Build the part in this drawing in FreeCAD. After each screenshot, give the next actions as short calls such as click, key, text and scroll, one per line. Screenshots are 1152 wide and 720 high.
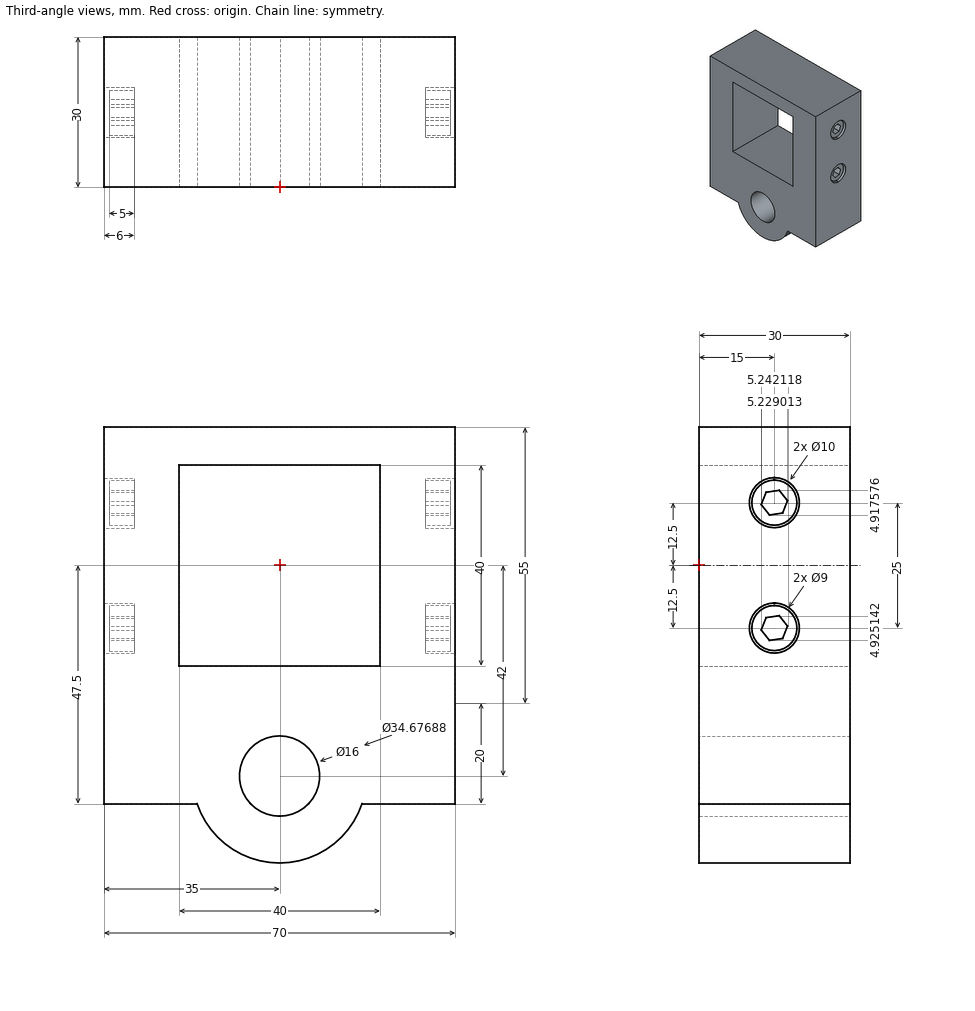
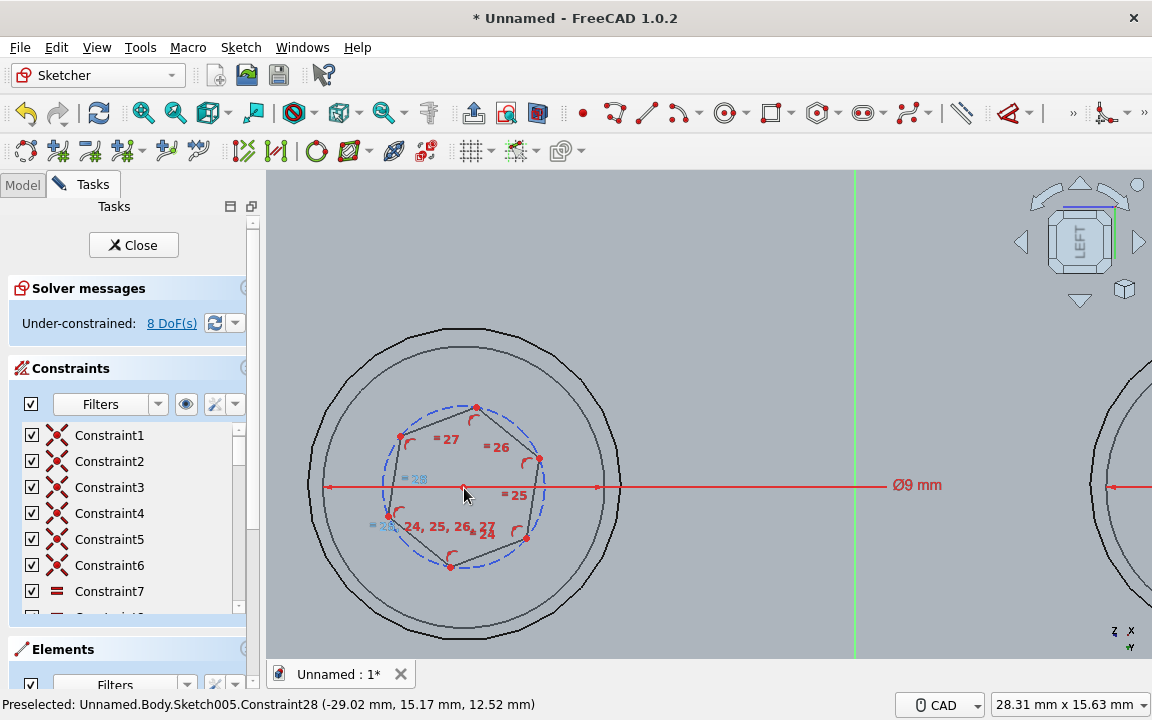
click(464, 487)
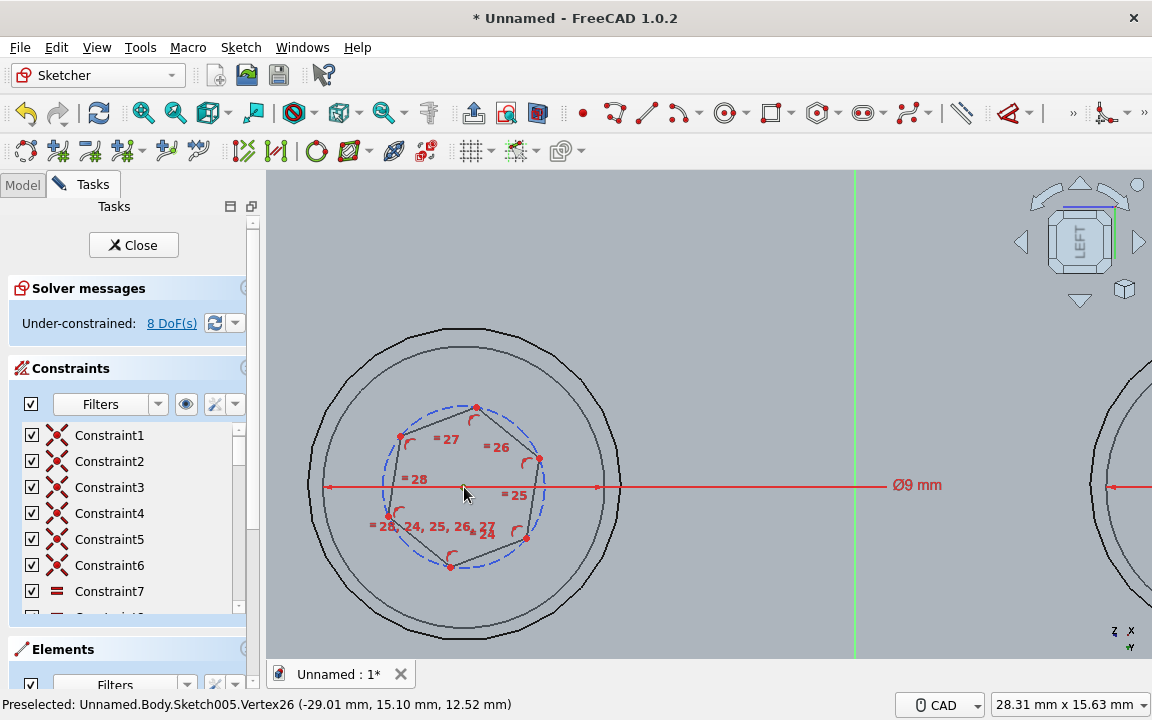
click(855, 600)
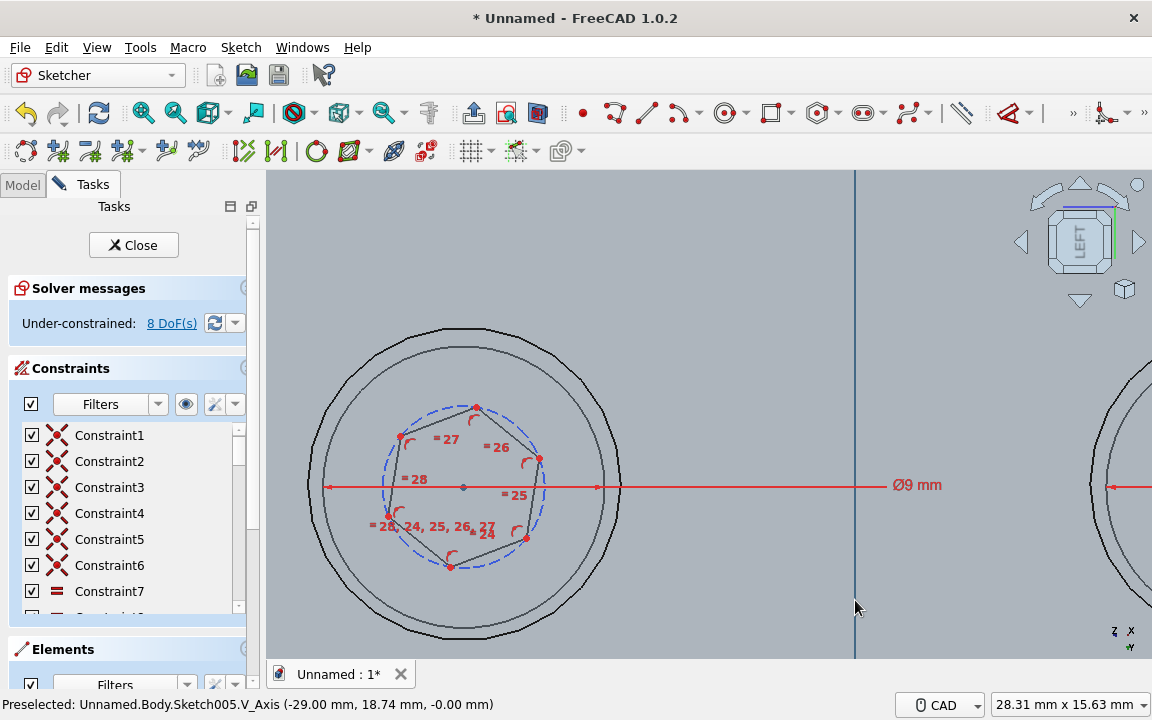
key(s)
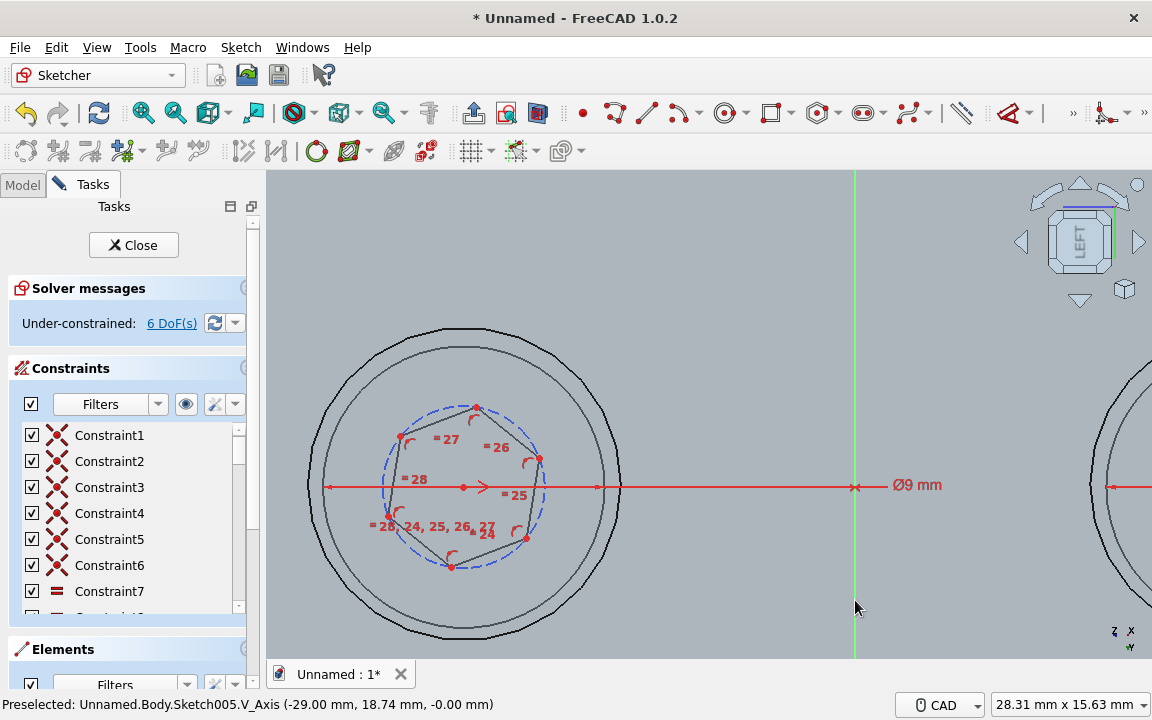
key(d)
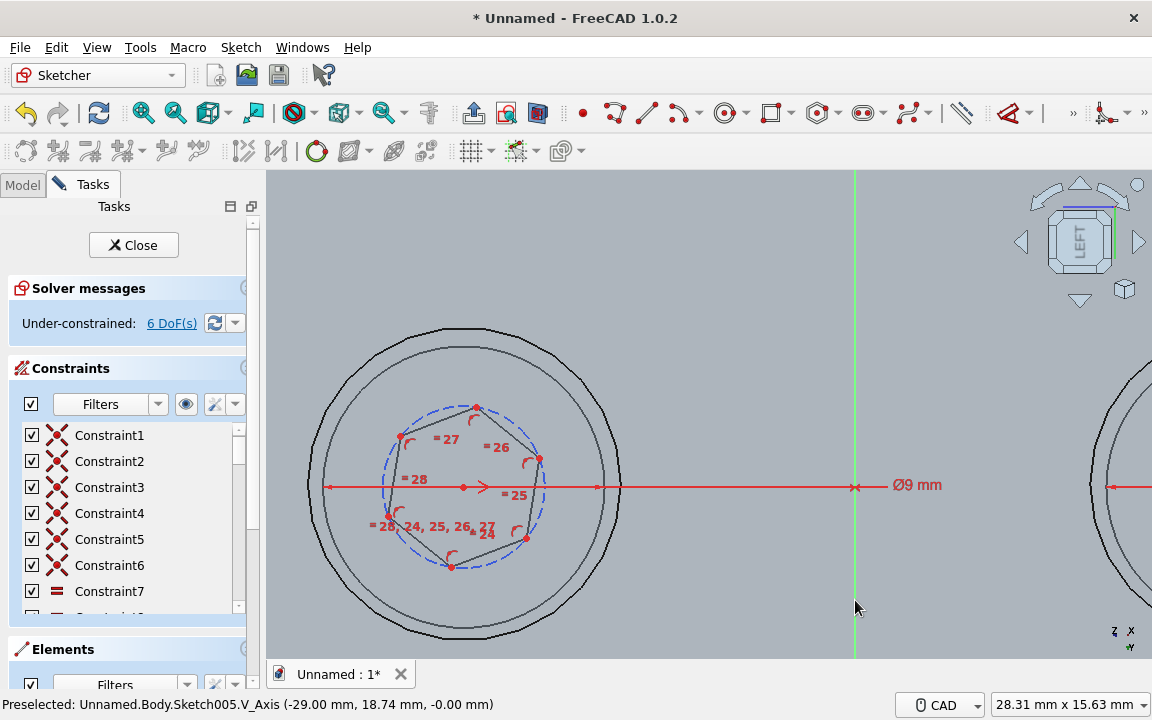
scroll(465, 492, down, 4)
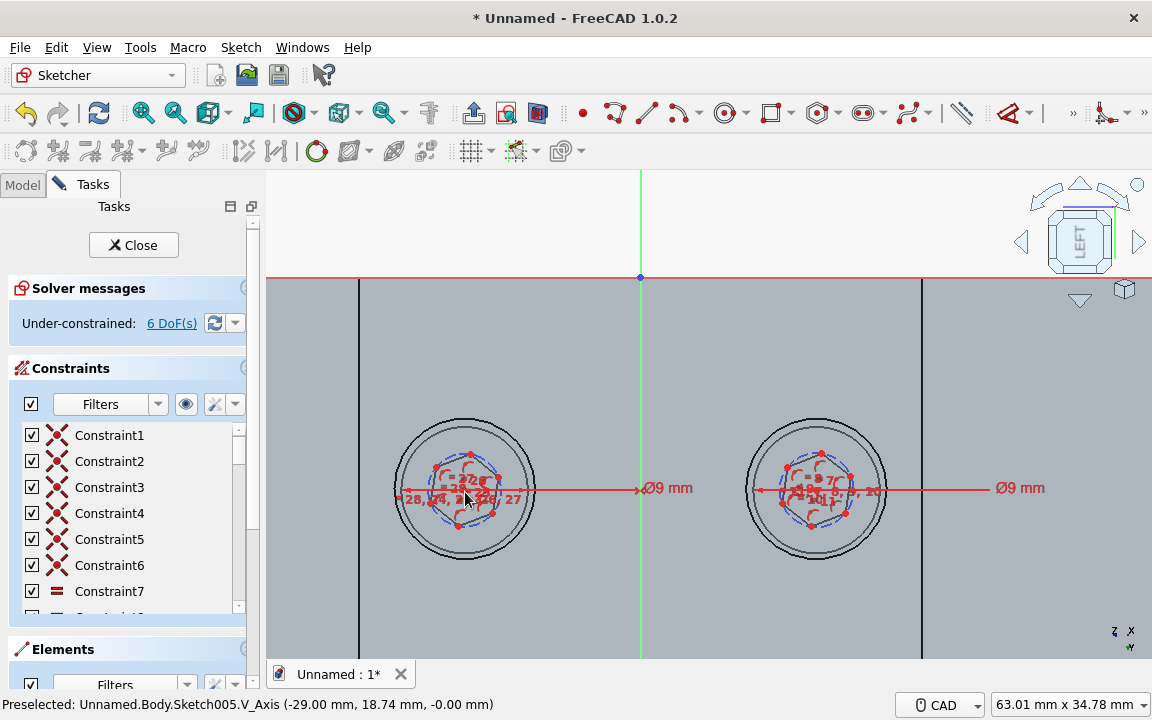
click(817, 490)
click(851, 384)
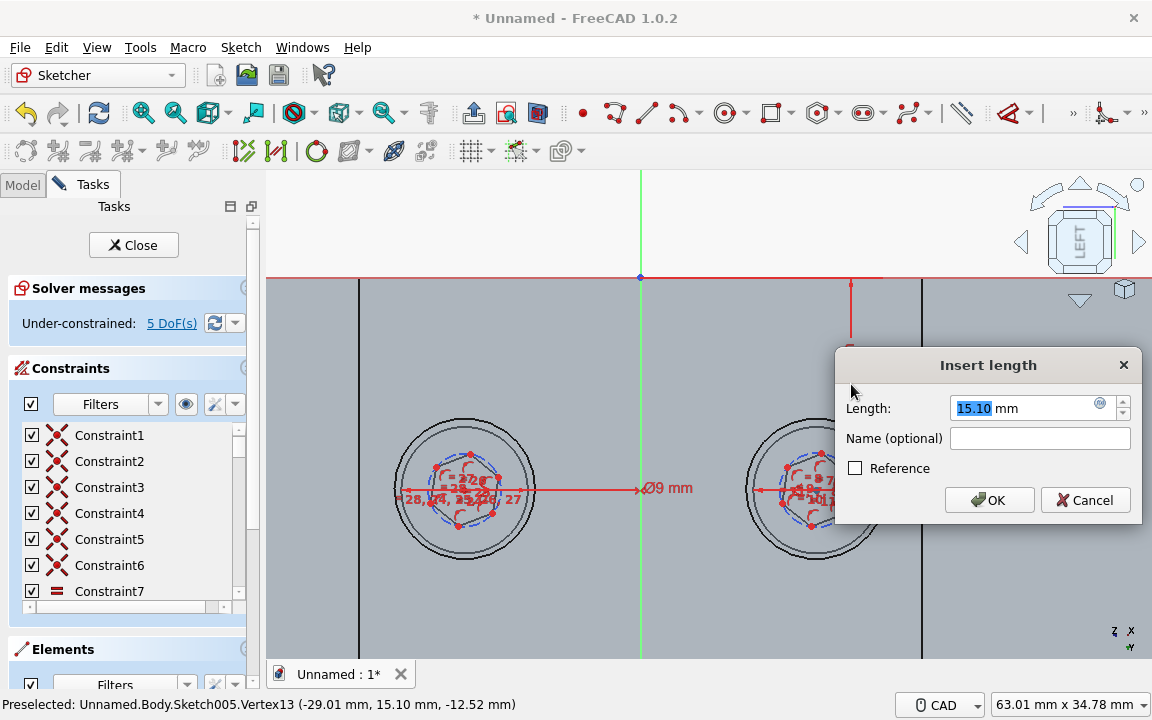
text(15)
key(Return)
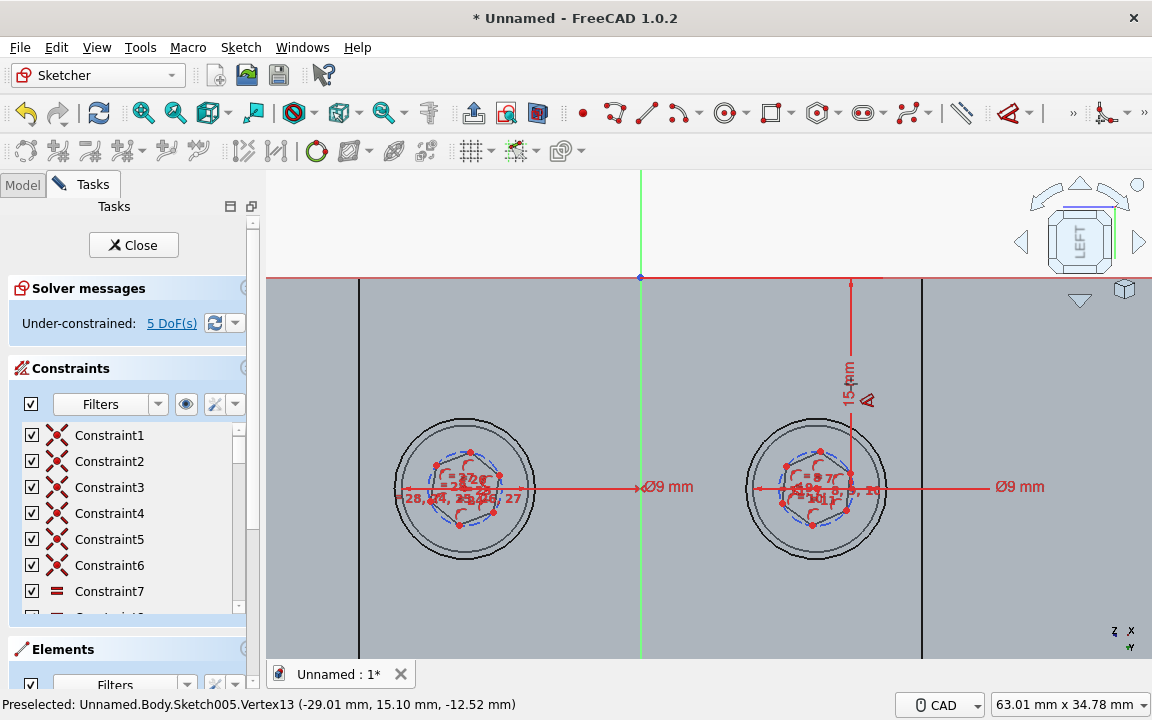
click(816, 489)
click(728, 244)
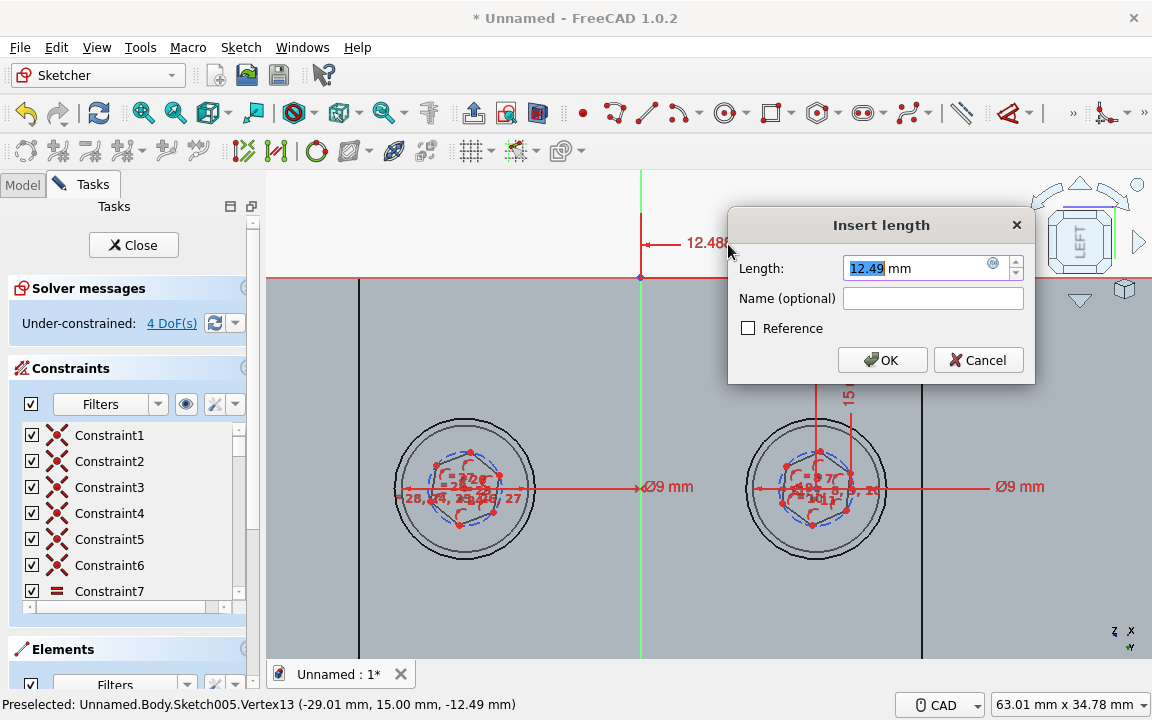
text(12.5)
key(Return)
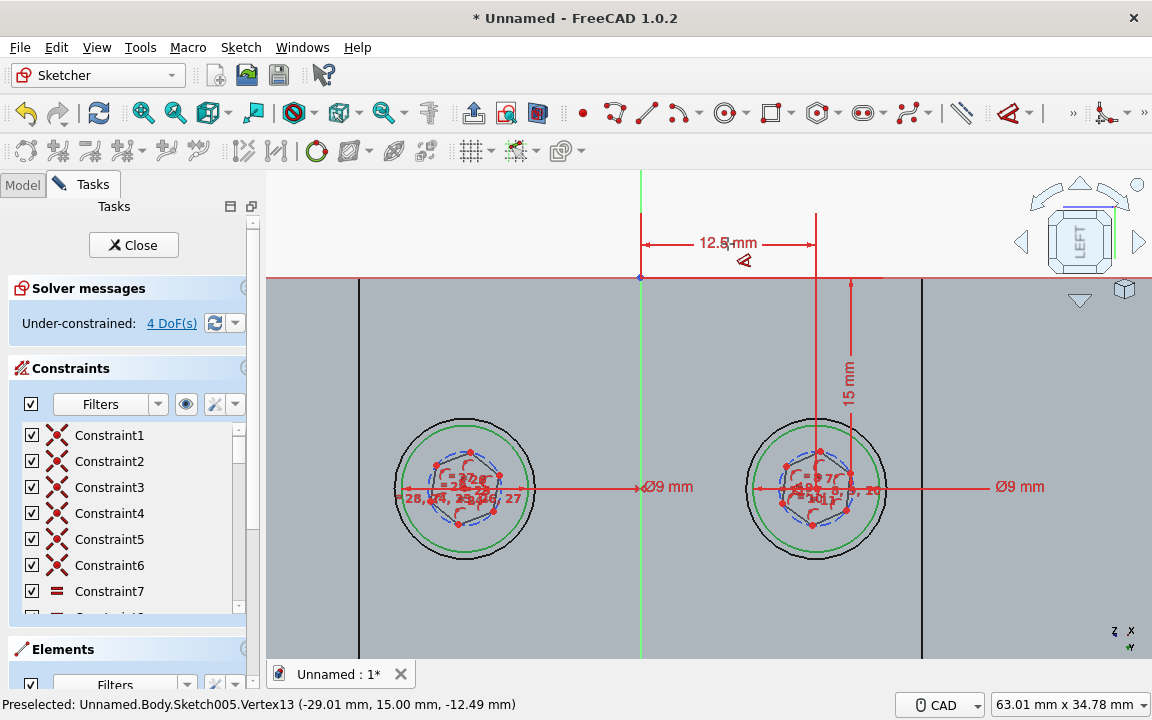
click(782, 504)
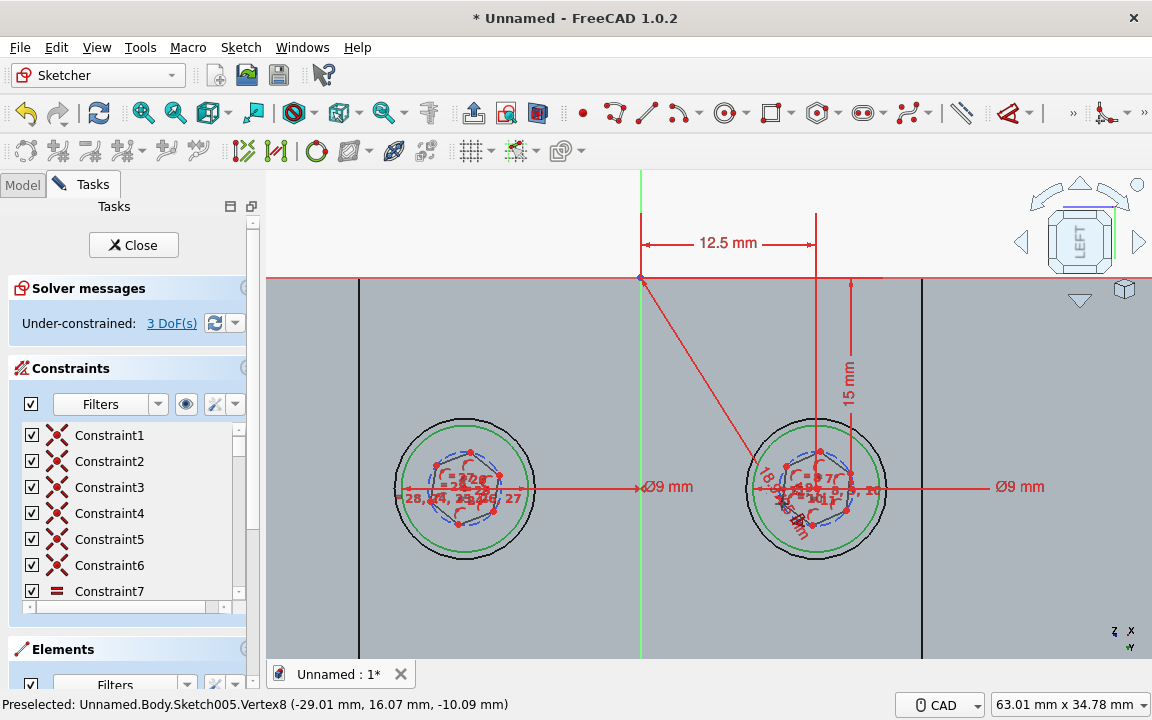
click(850, 474)
click(793, 562)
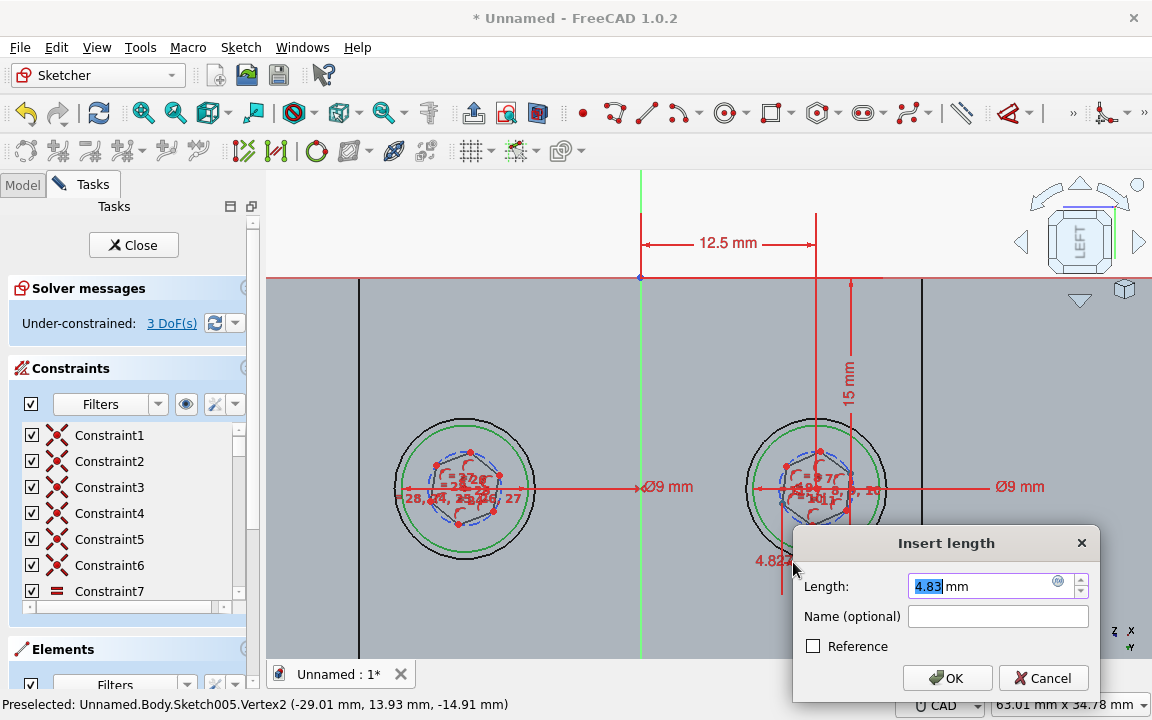
text(4.925142)
key(Return)